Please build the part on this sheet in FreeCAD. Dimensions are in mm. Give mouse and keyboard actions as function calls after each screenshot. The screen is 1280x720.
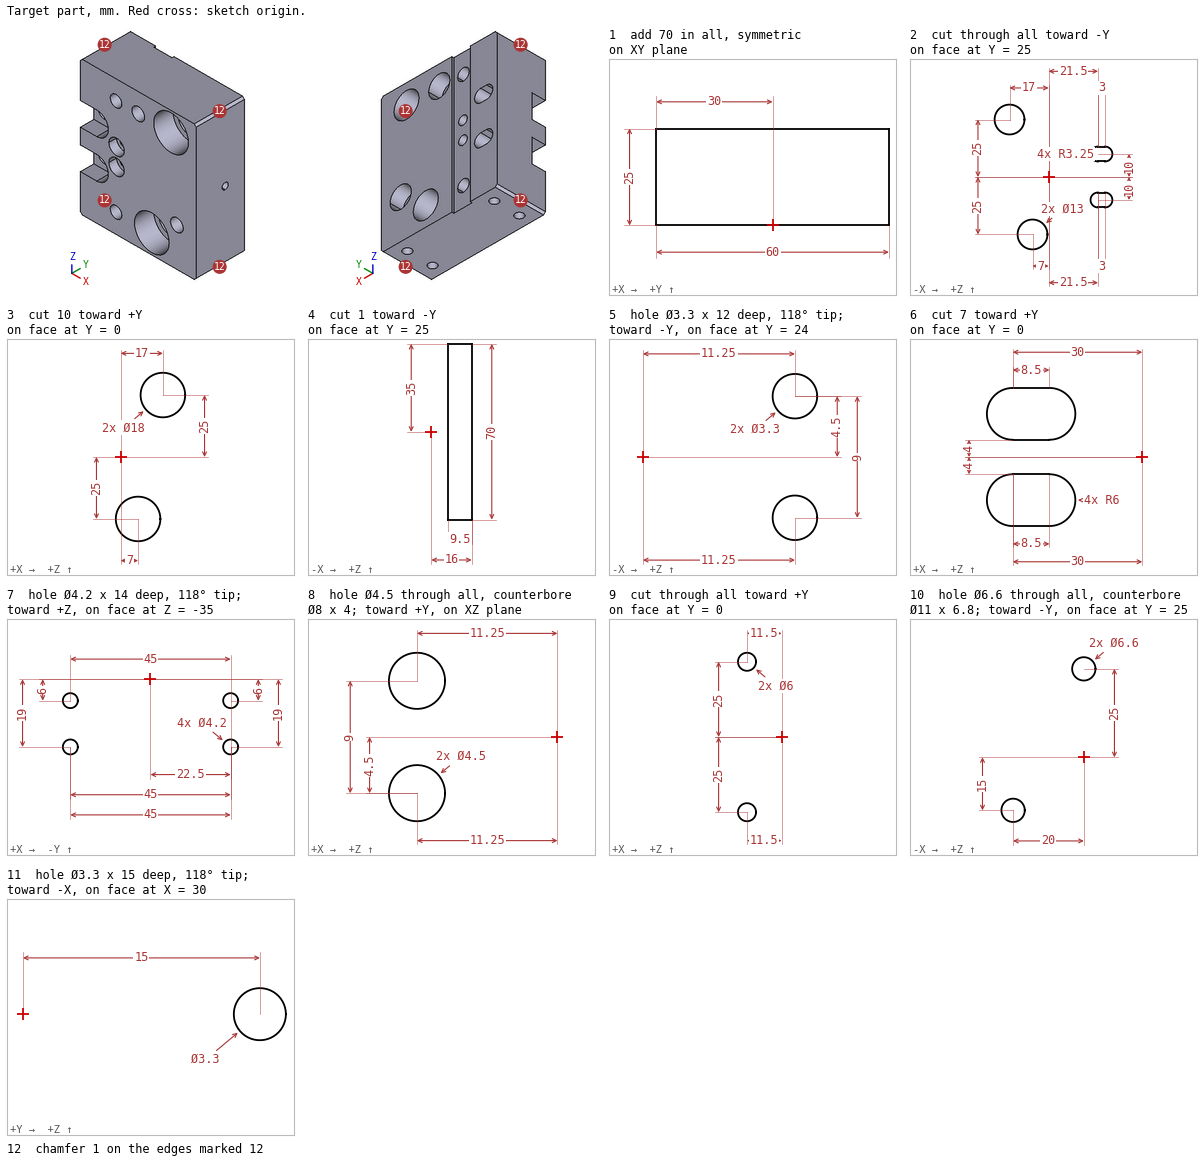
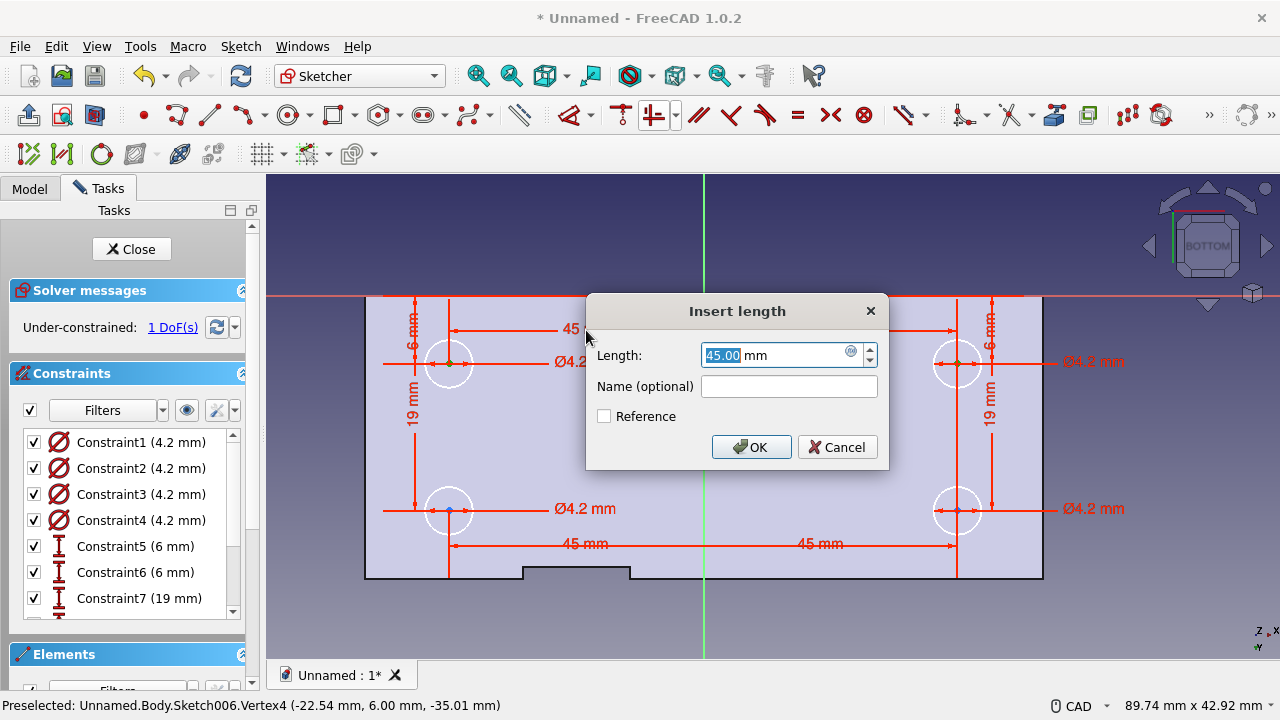
text(45)
key(Return)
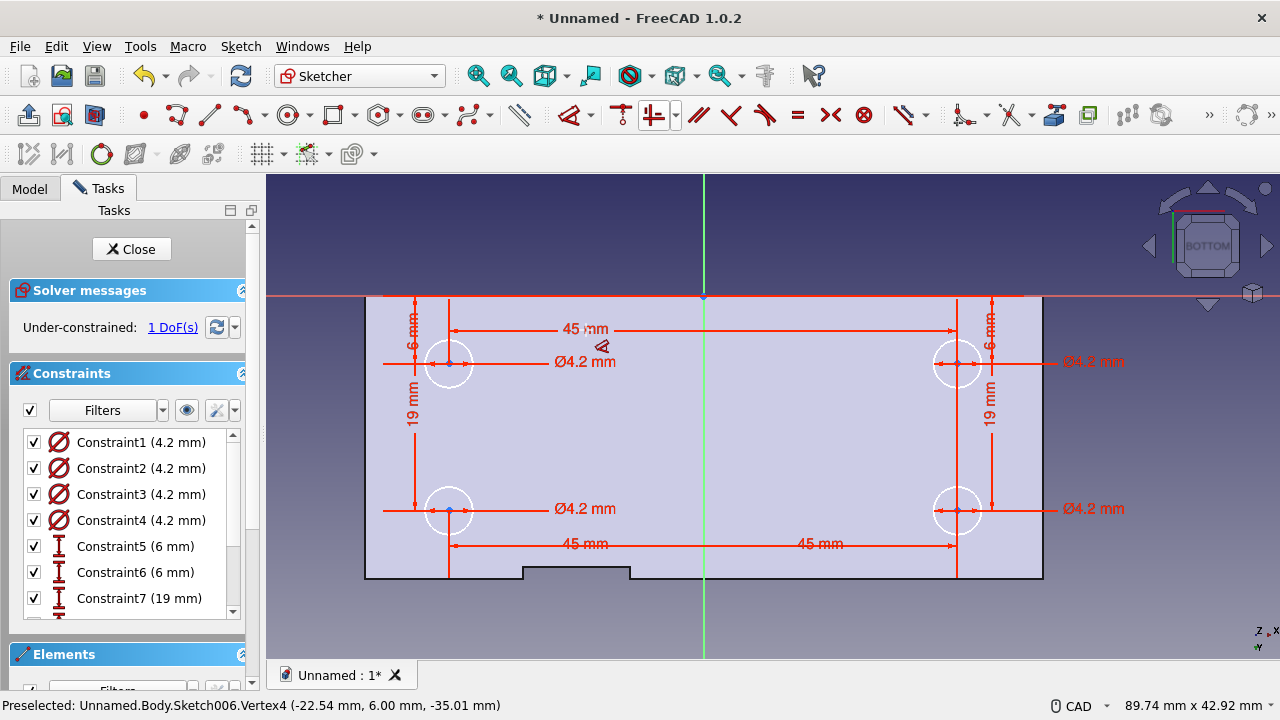
click(957, 511)
click(831, 262)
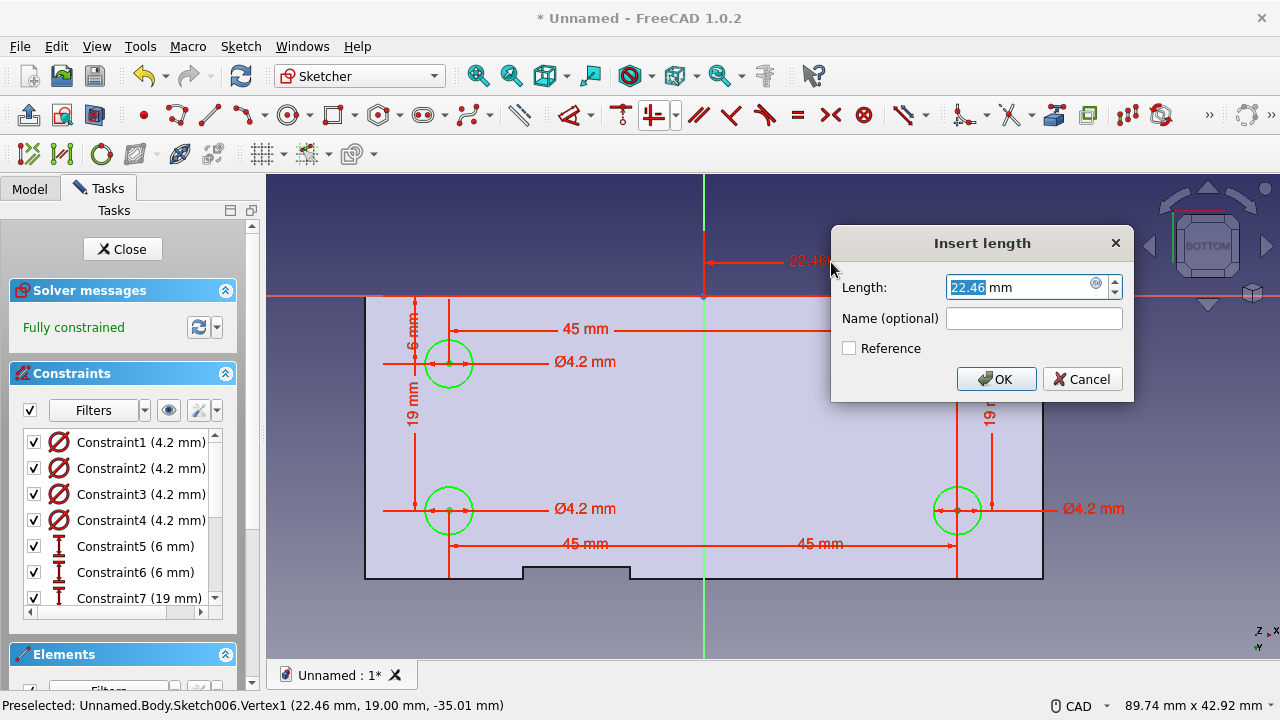
text(22.5)
key(Return)
key(Escape)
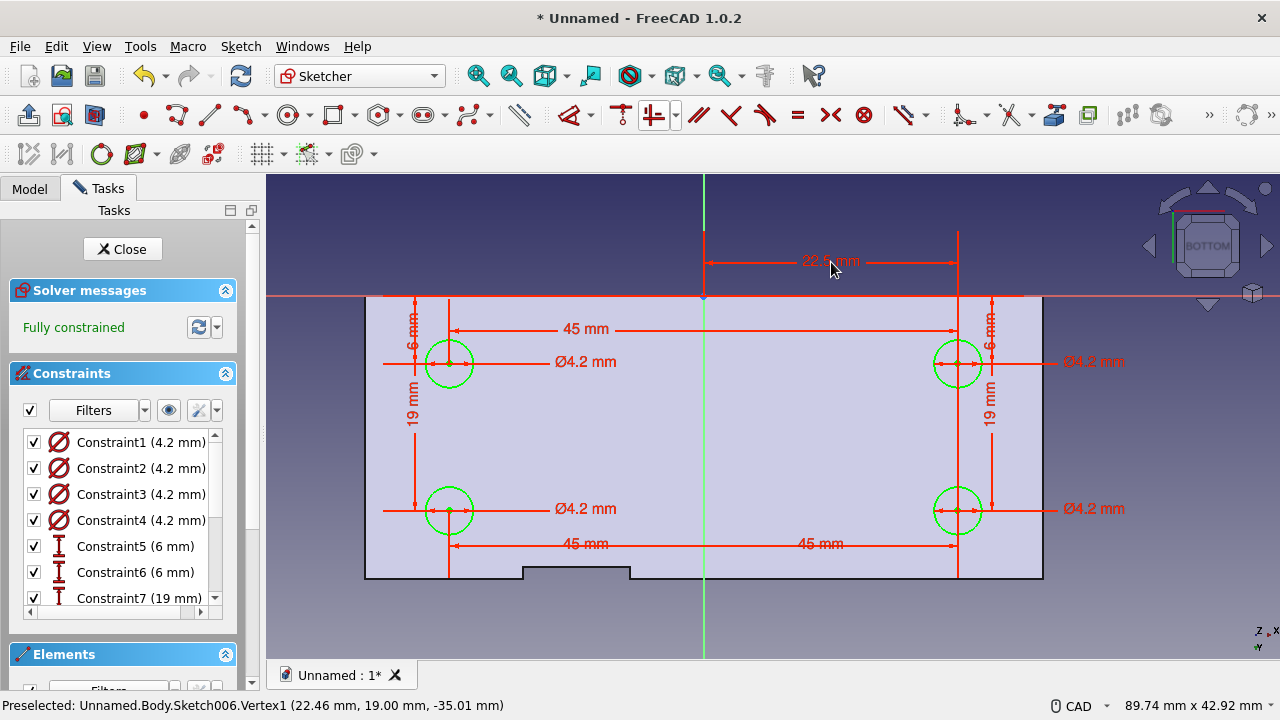
click(123, 249)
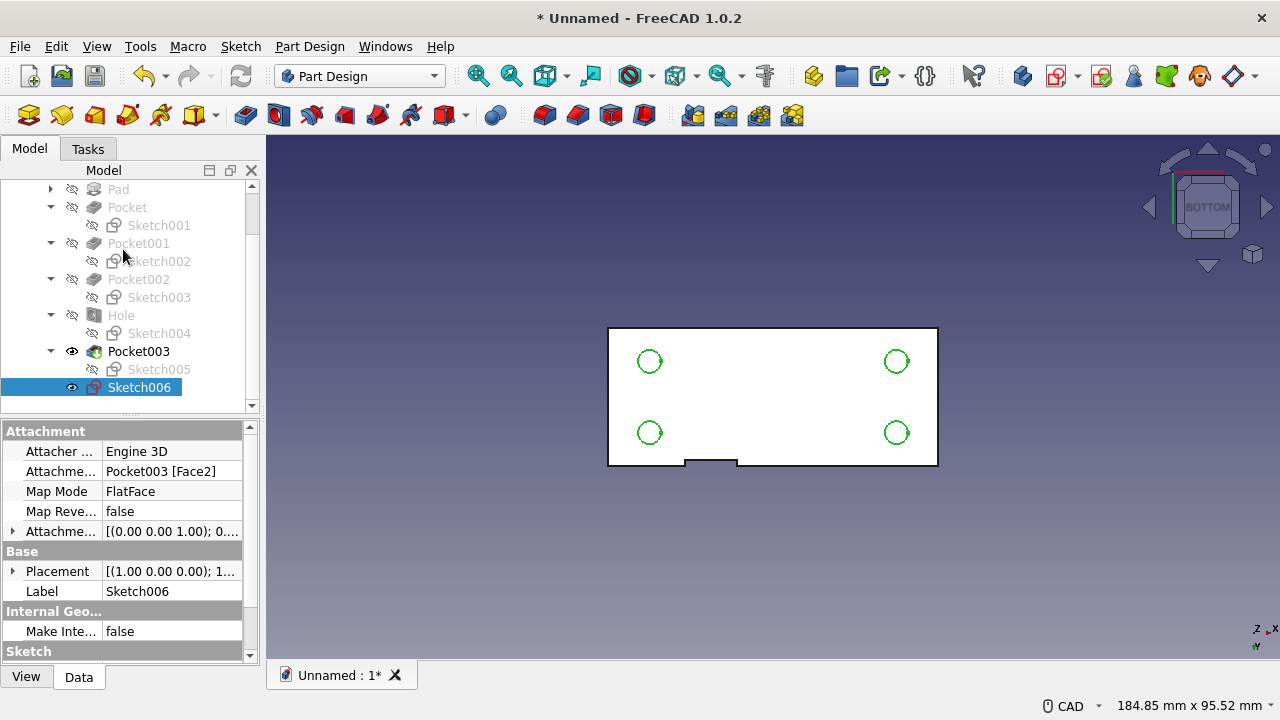
click(279, 116)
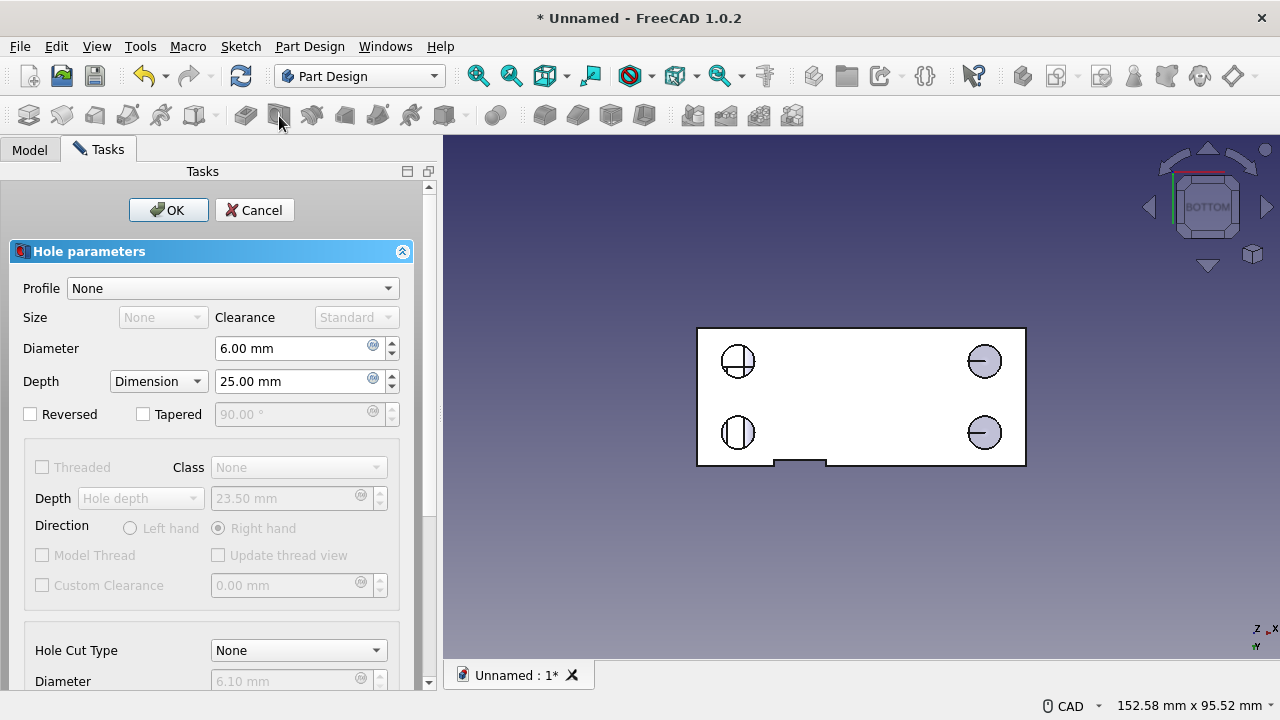
triple_click(300, 348)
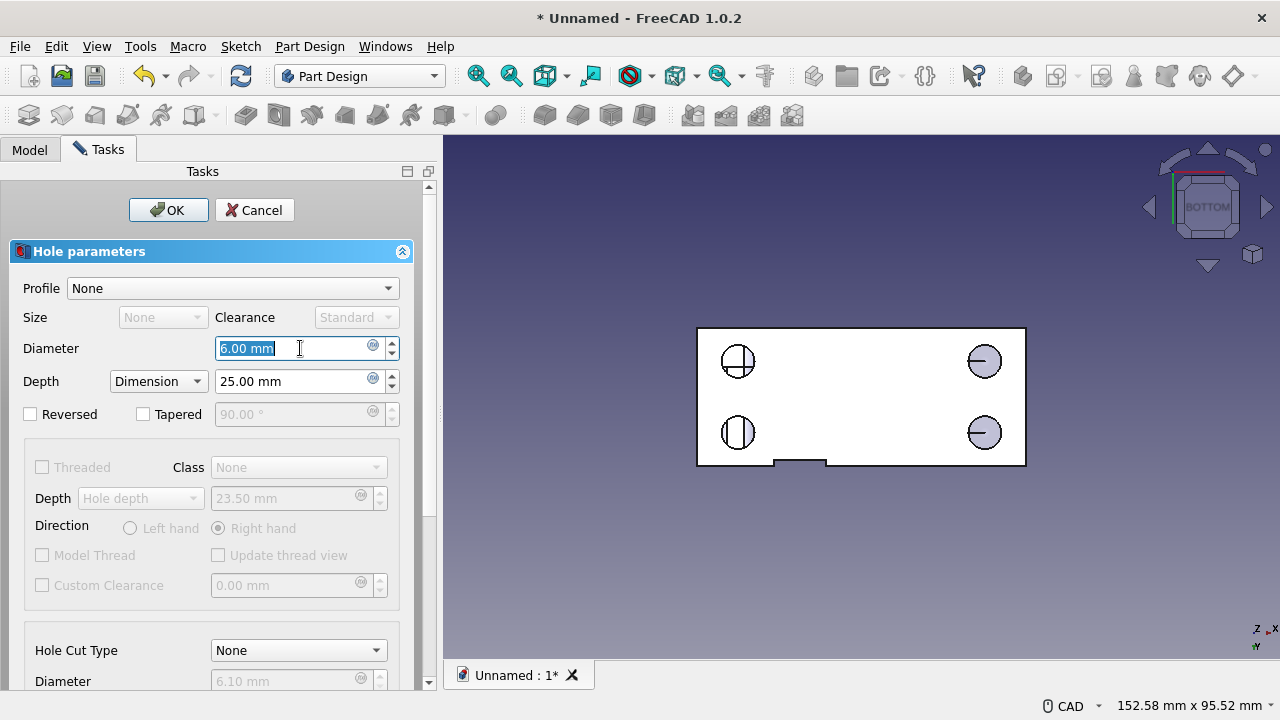
text(4.2)
key(Tab)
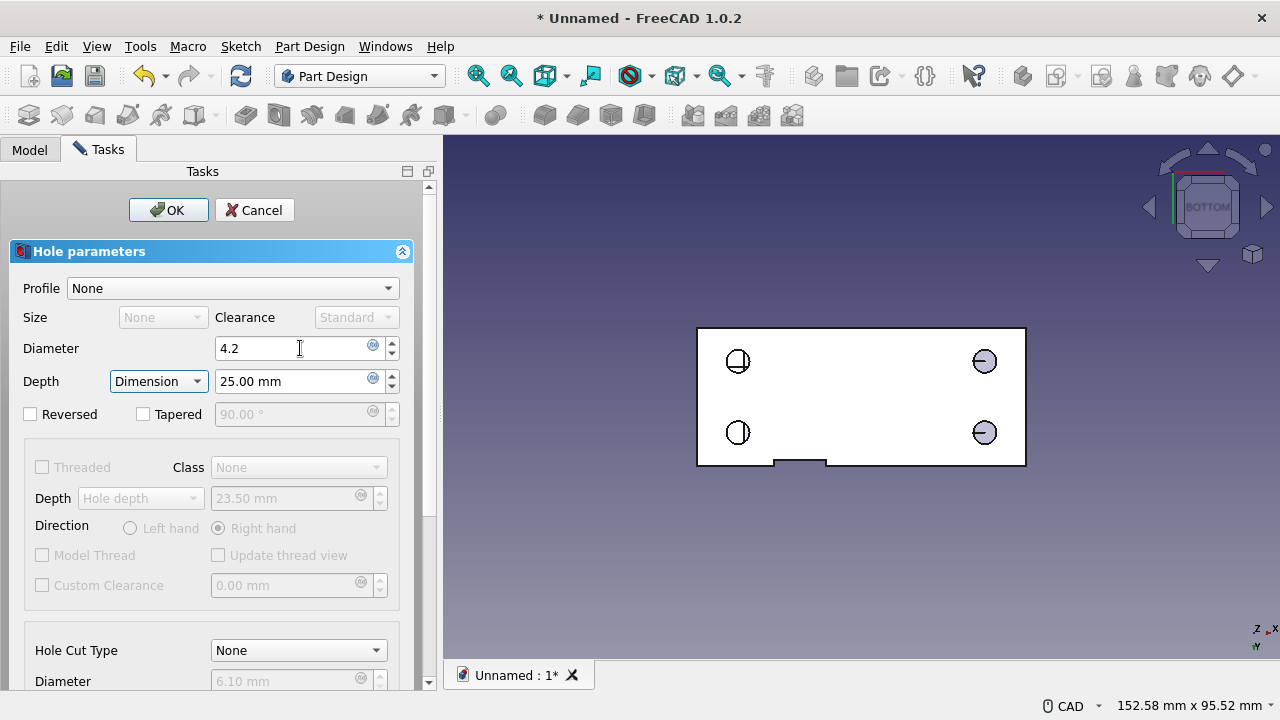
triple_click(300, 382)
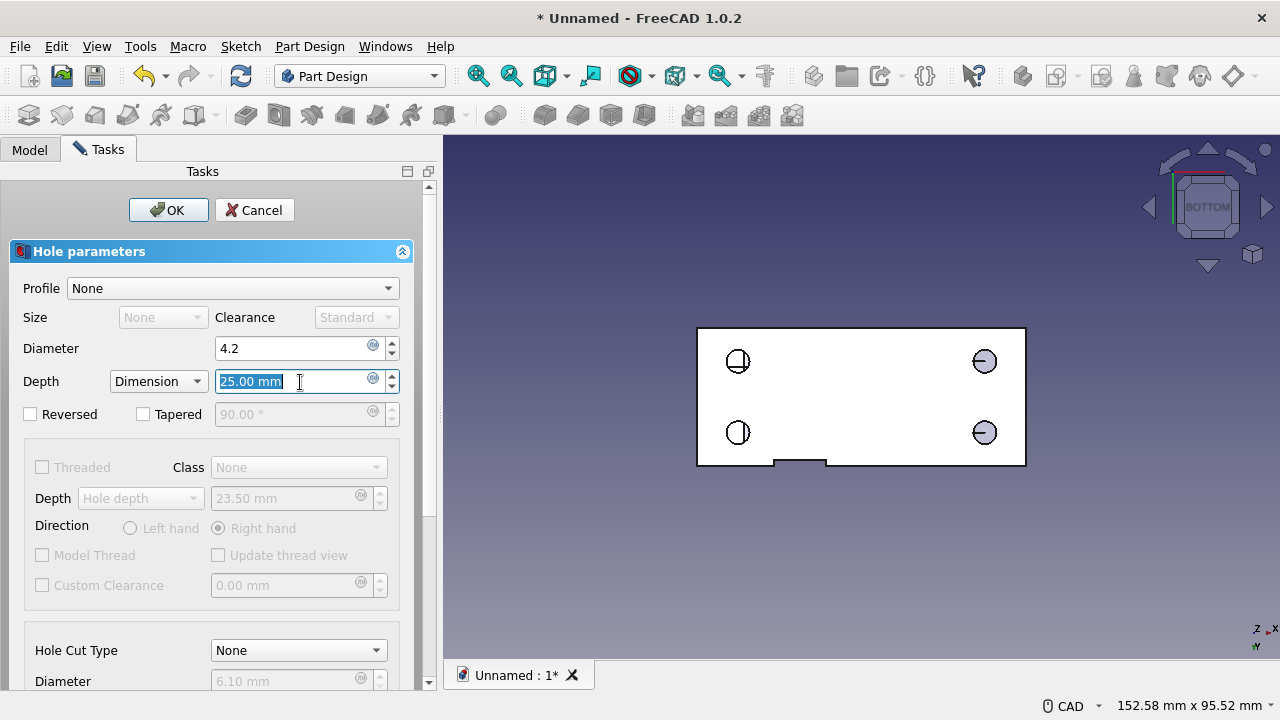
text(14)
key(Tab)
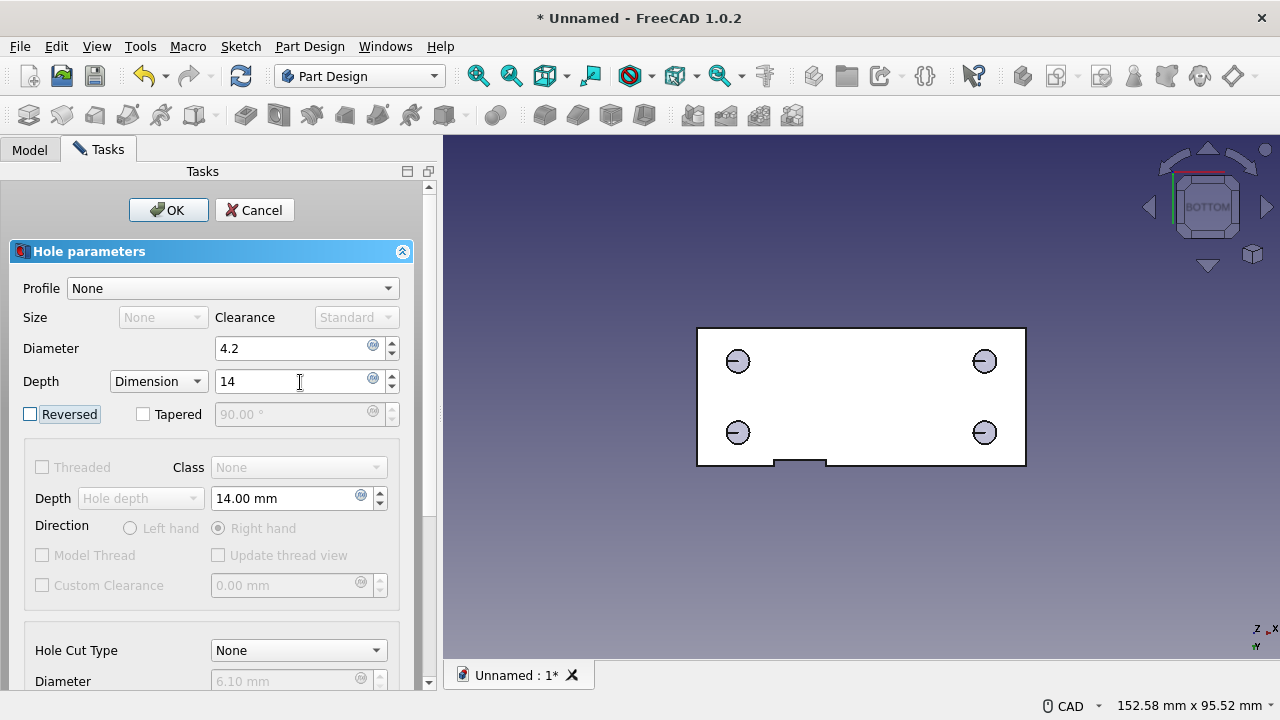
click(169, 210)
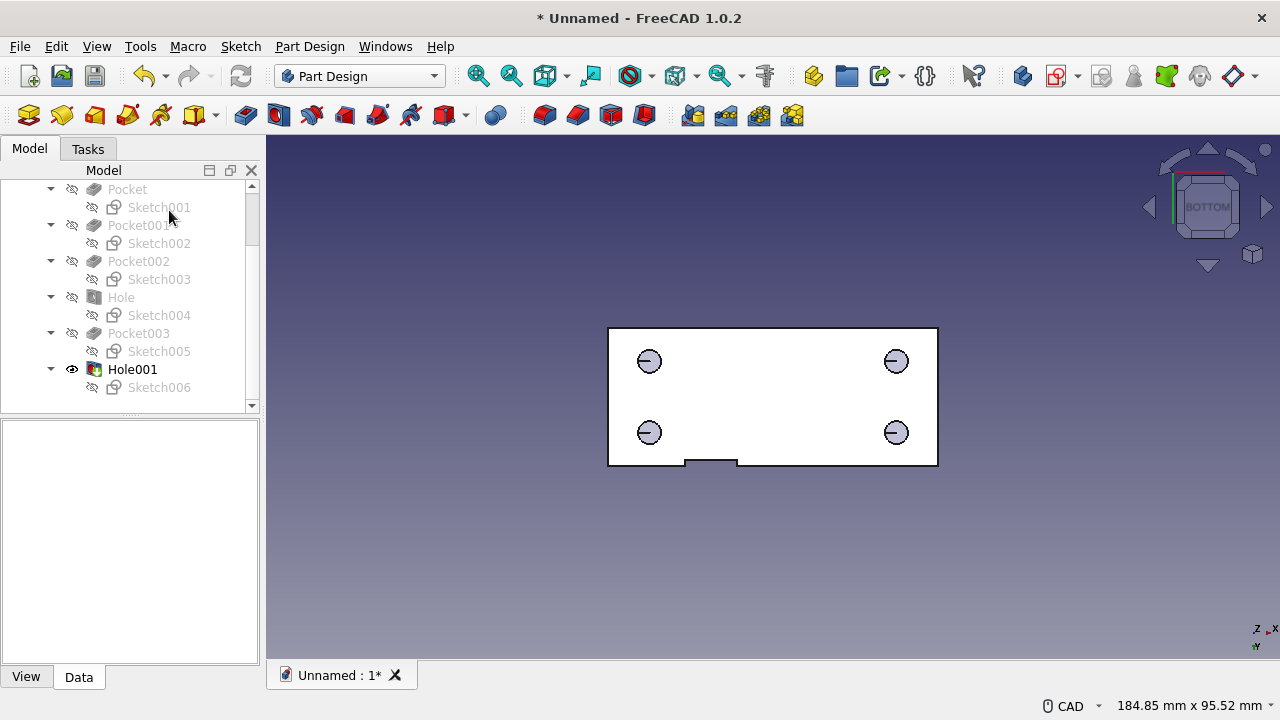
key(v)
key(f)